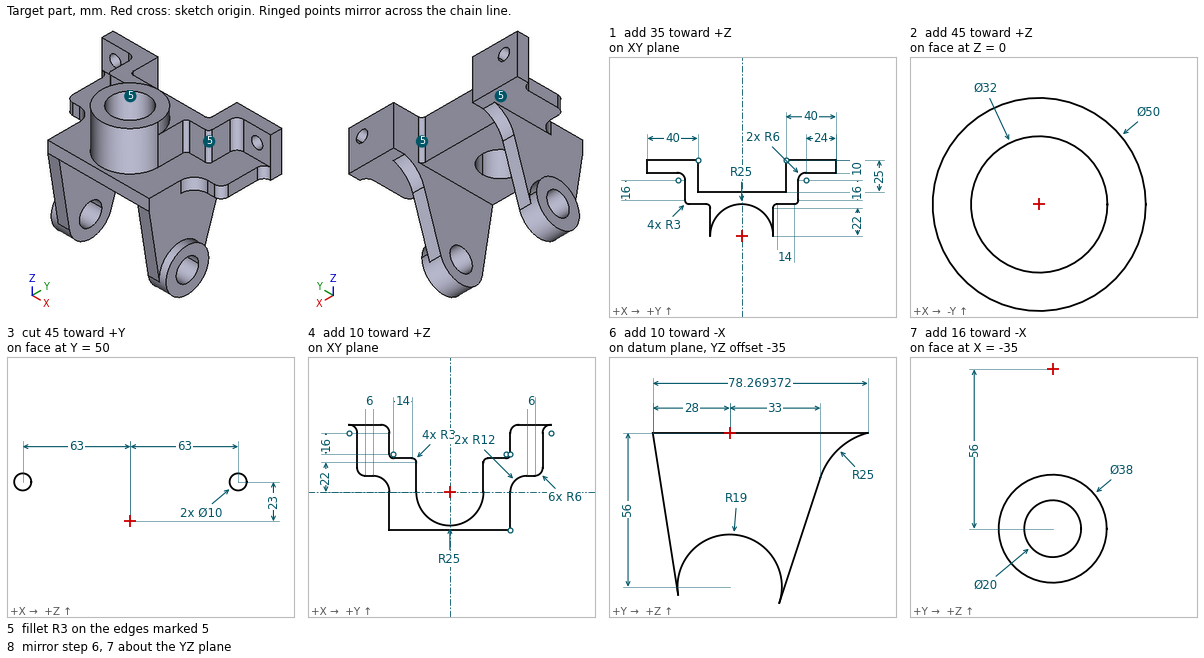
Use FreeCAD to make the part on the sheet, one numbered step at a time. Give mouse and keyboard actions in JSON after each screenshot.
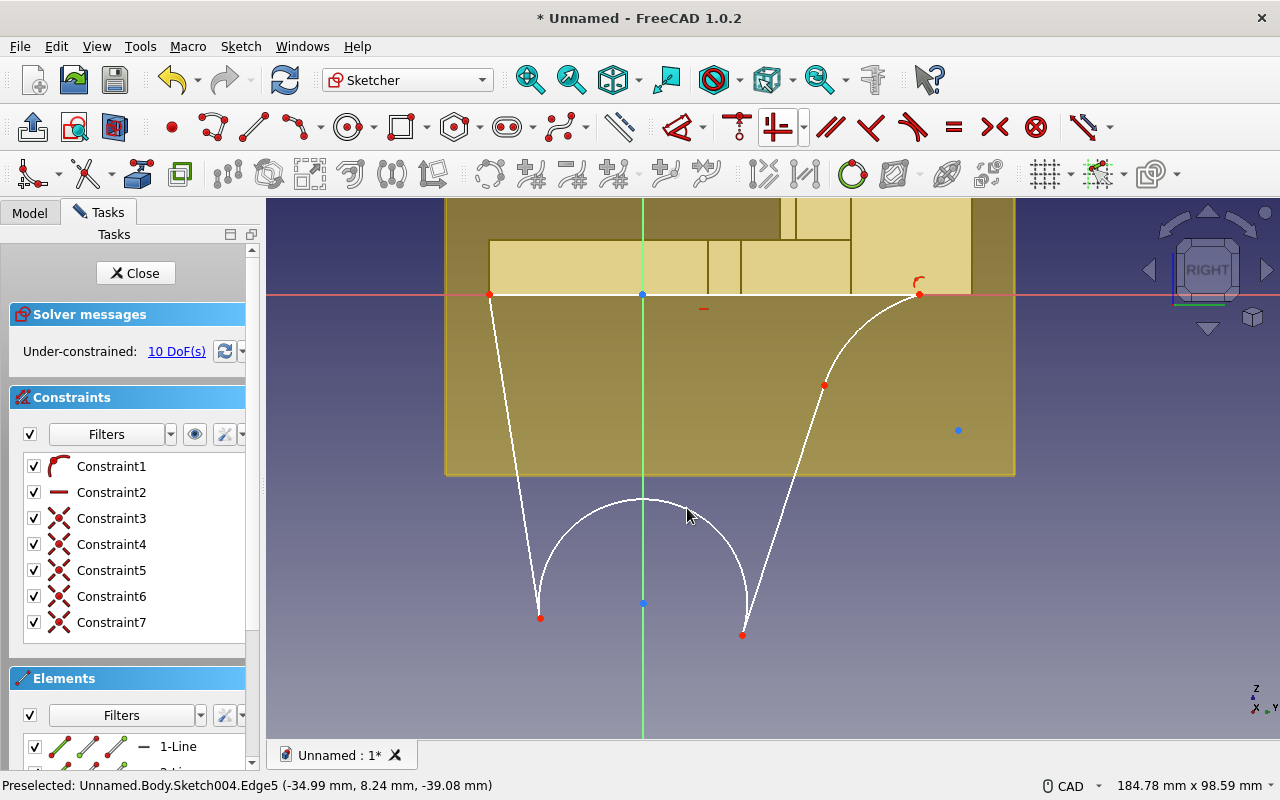
{"action": "left_click", "coordinate": [767, 561]}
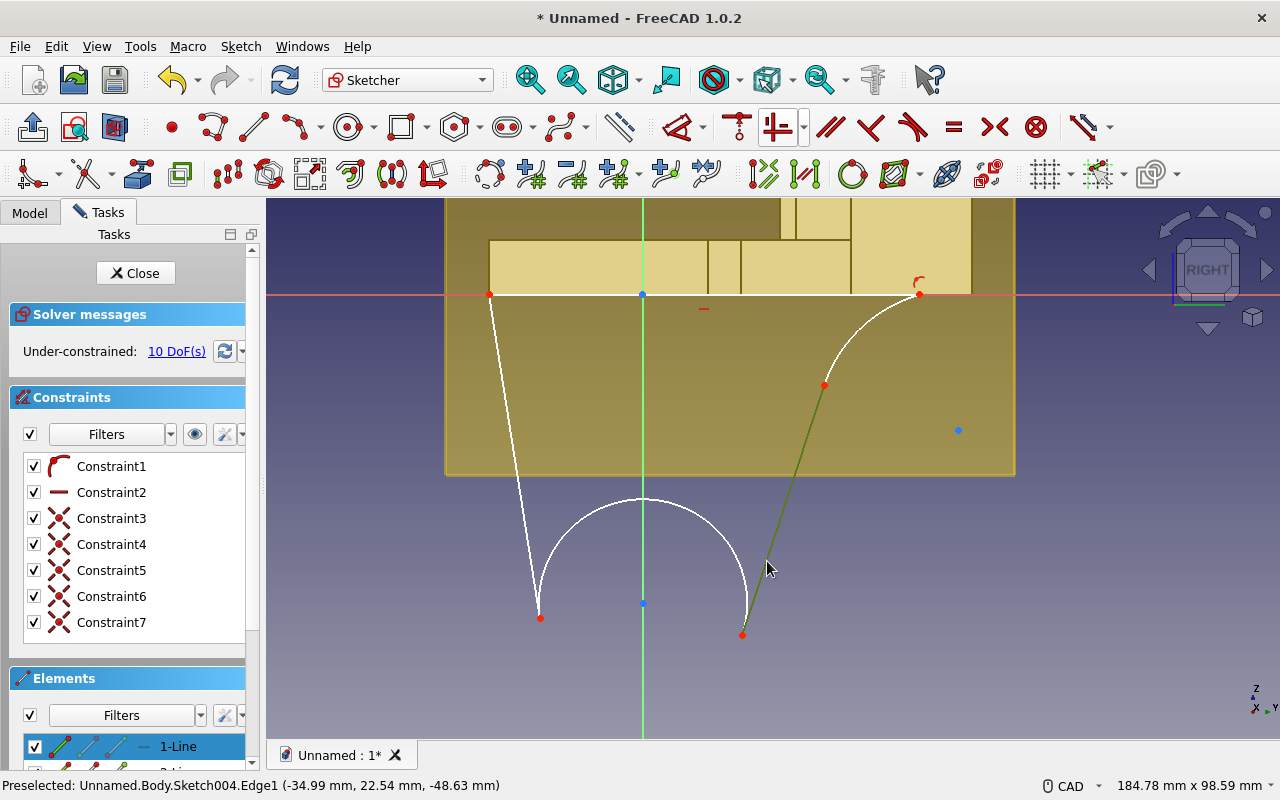
{"action": "left_click", "coordinate": [882, 312]}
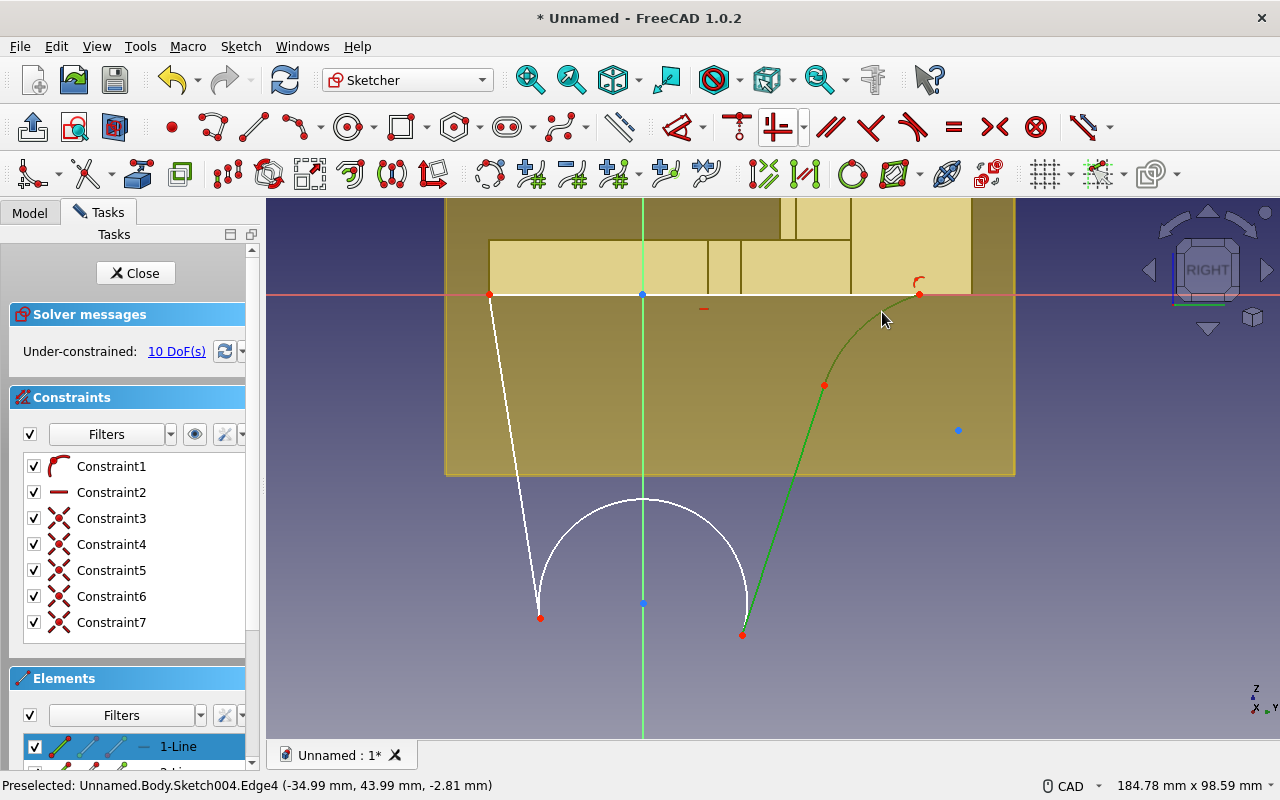
{"action": "left_click", "coordinate": [913, 128]}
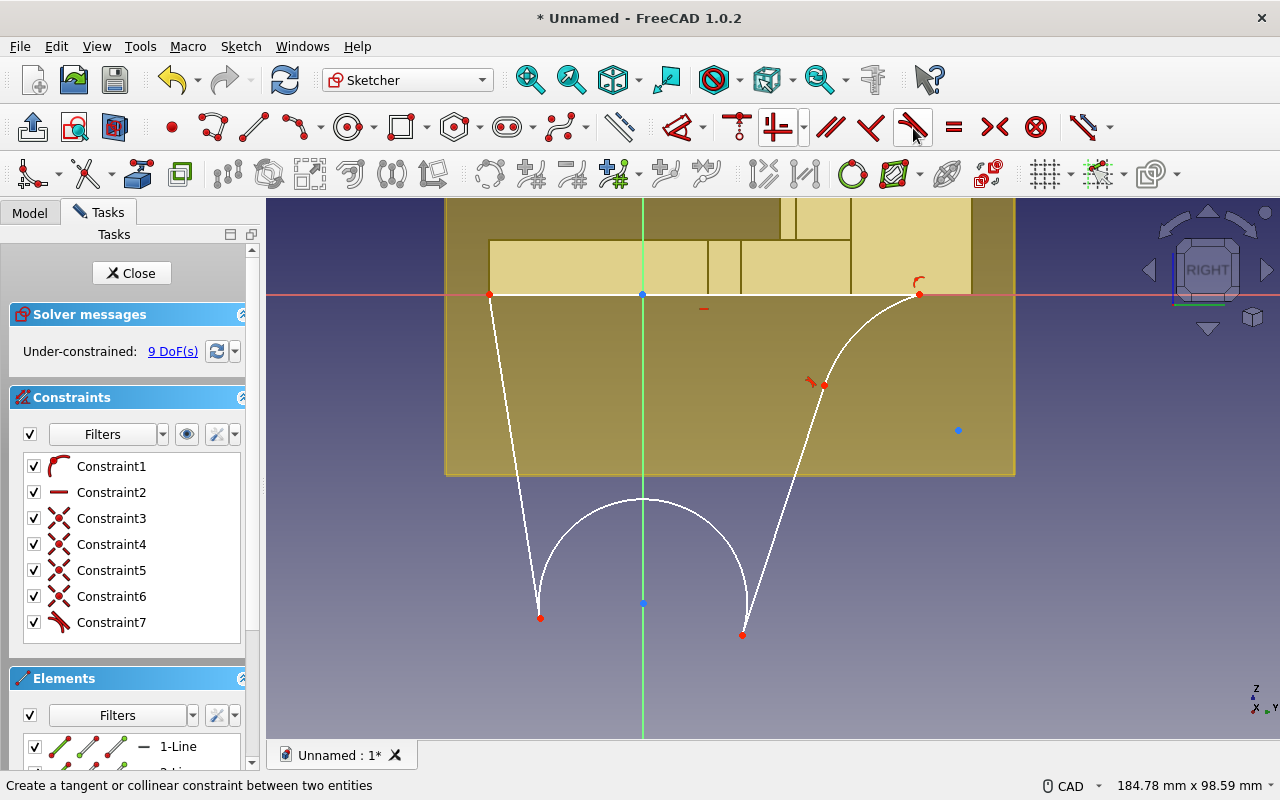
{"action": "left_click", "coordinate": [767, 561]}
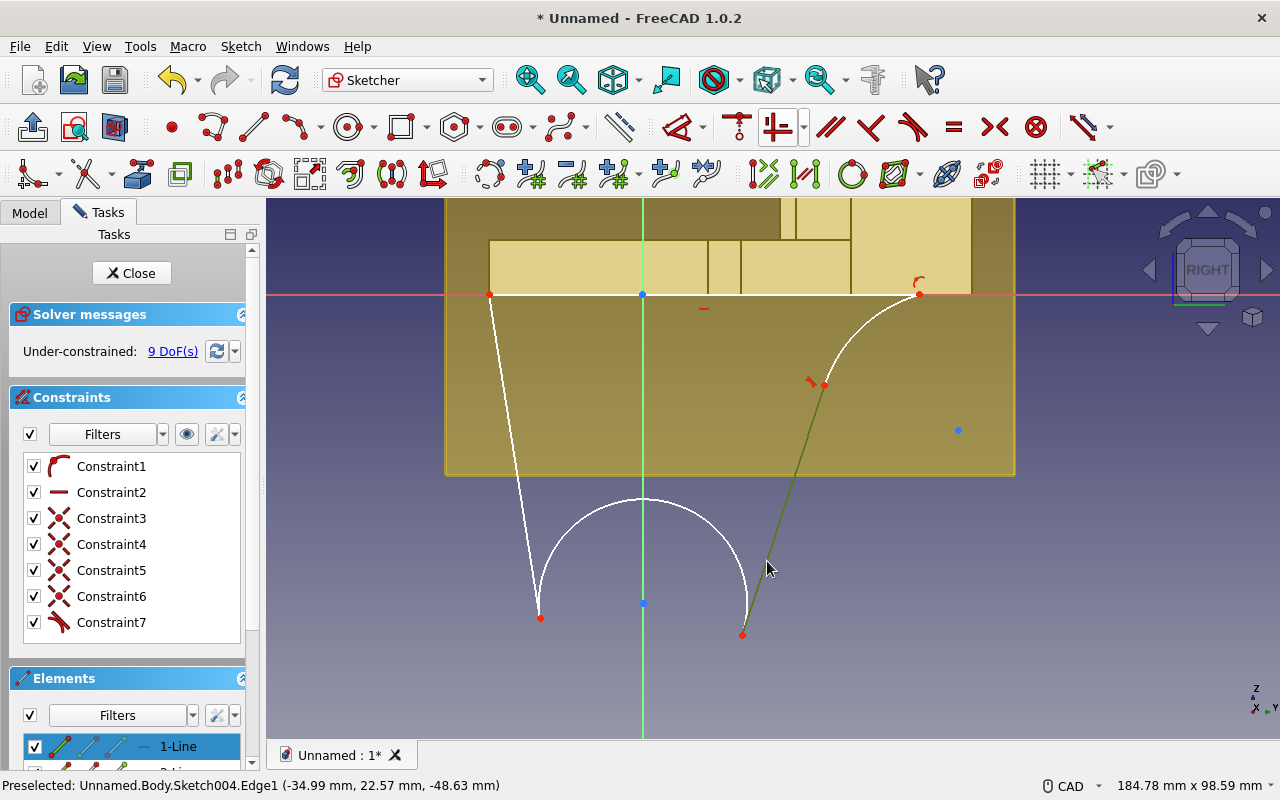
{"action": "left_click", "coordinate": [718, 531]}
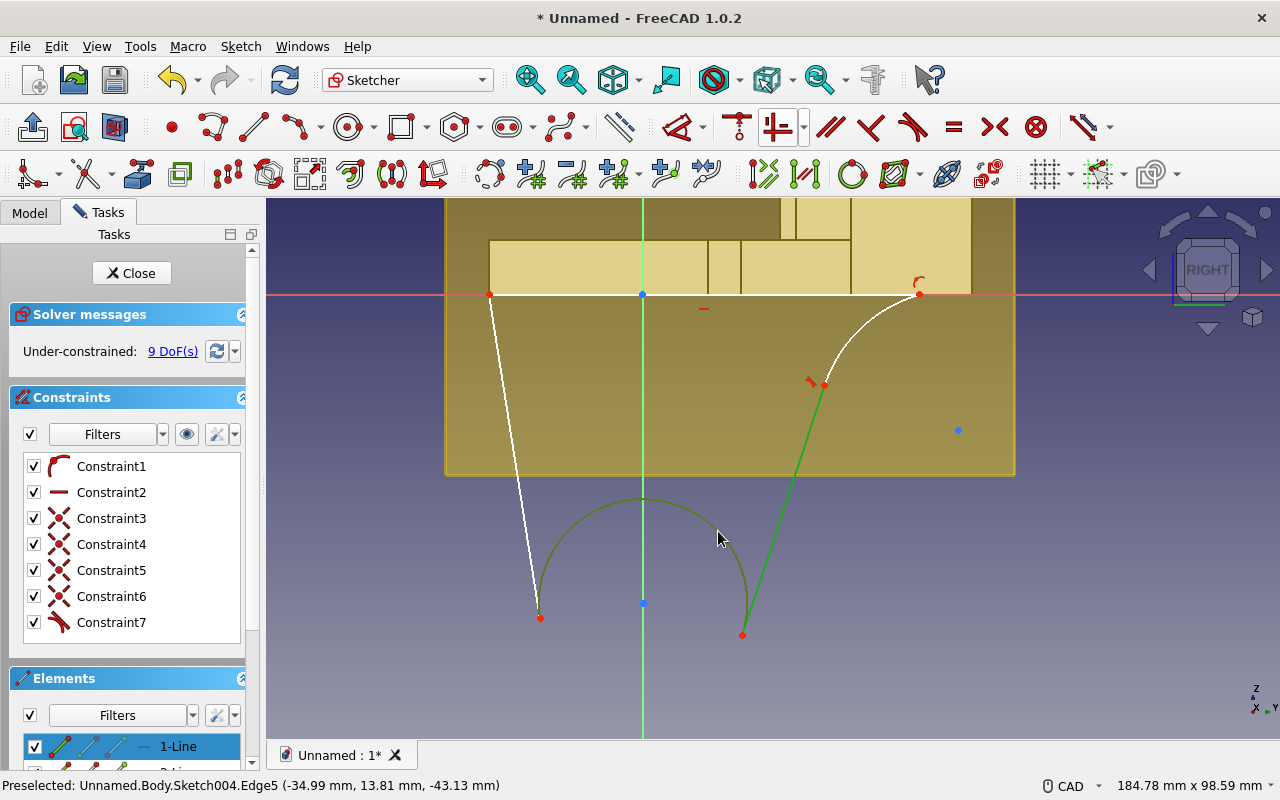
{"action": "left_click", "coordinate": [913, 128]}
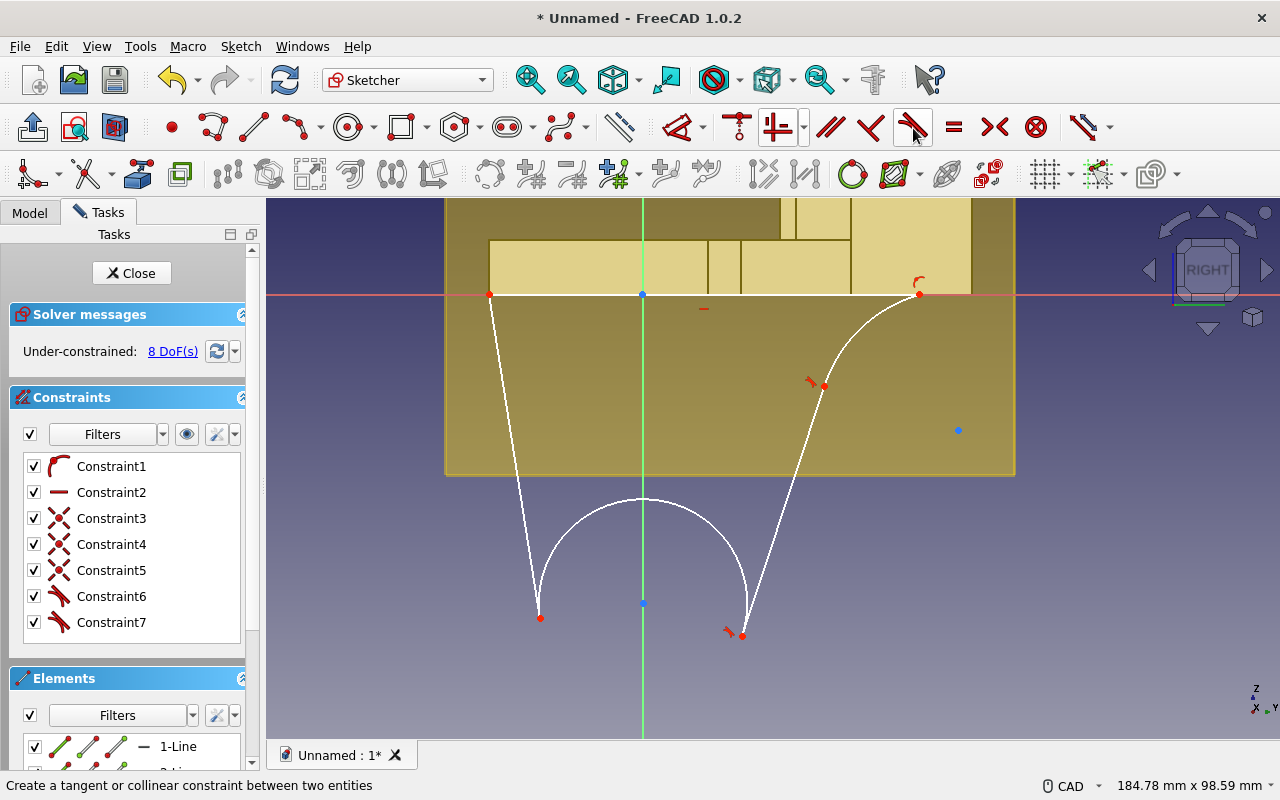
{"action": "left_click", "coordinate": [504, 392]}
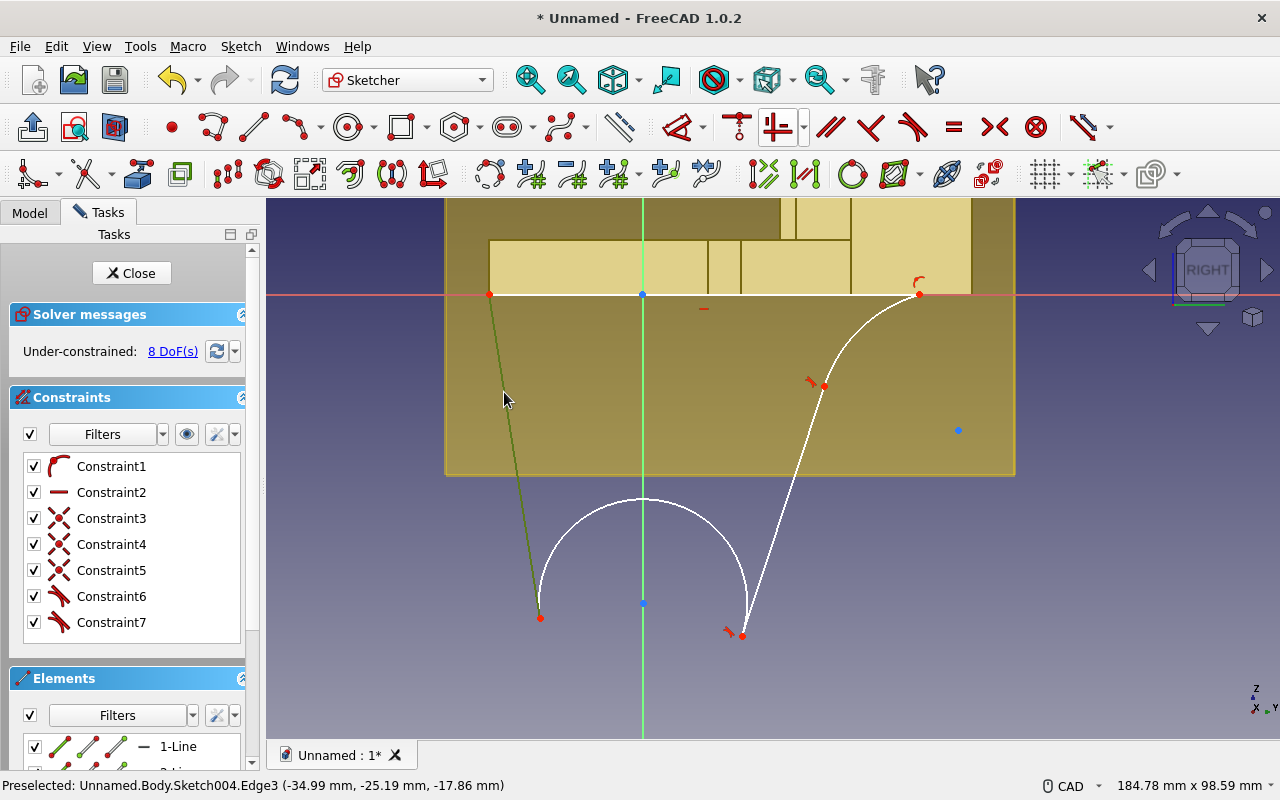
{"action": "left_click", "coordinate": [718, 531]}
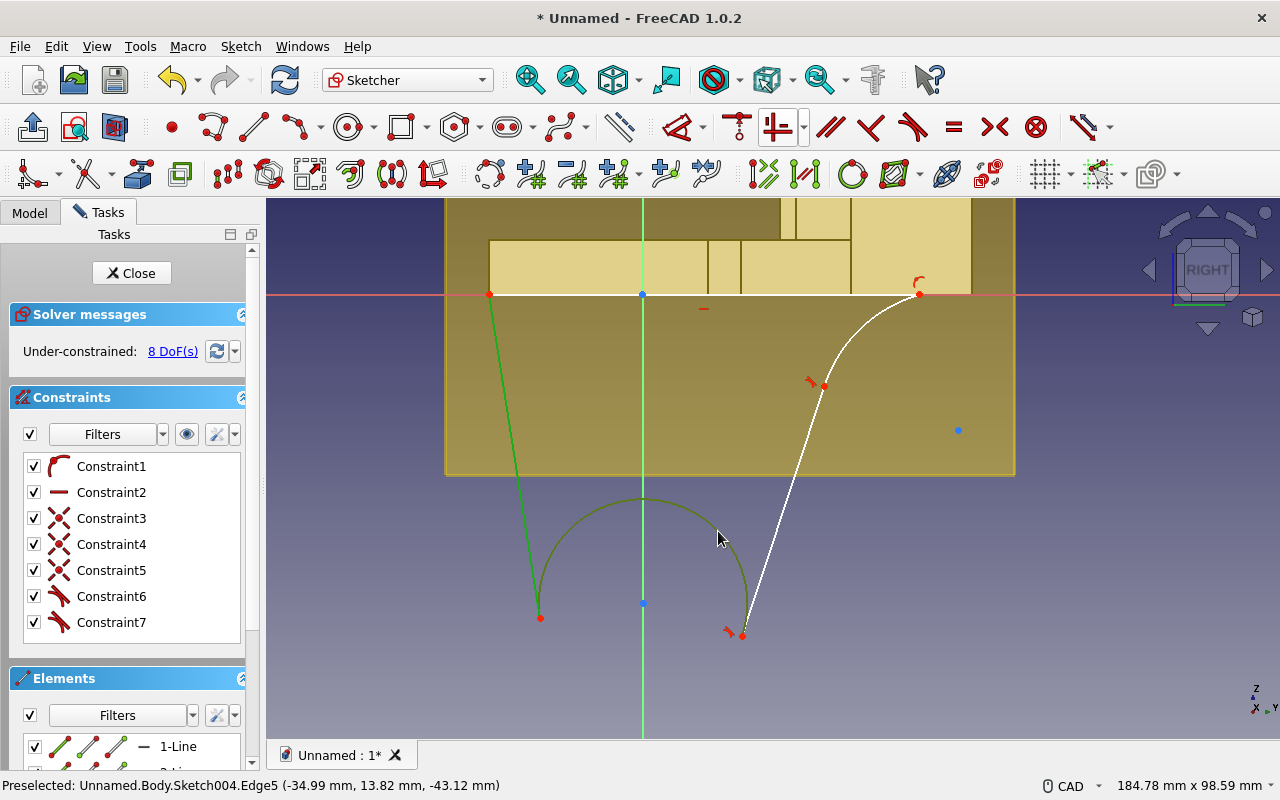
{"action": "left_click", "coordinate": [913, 128]}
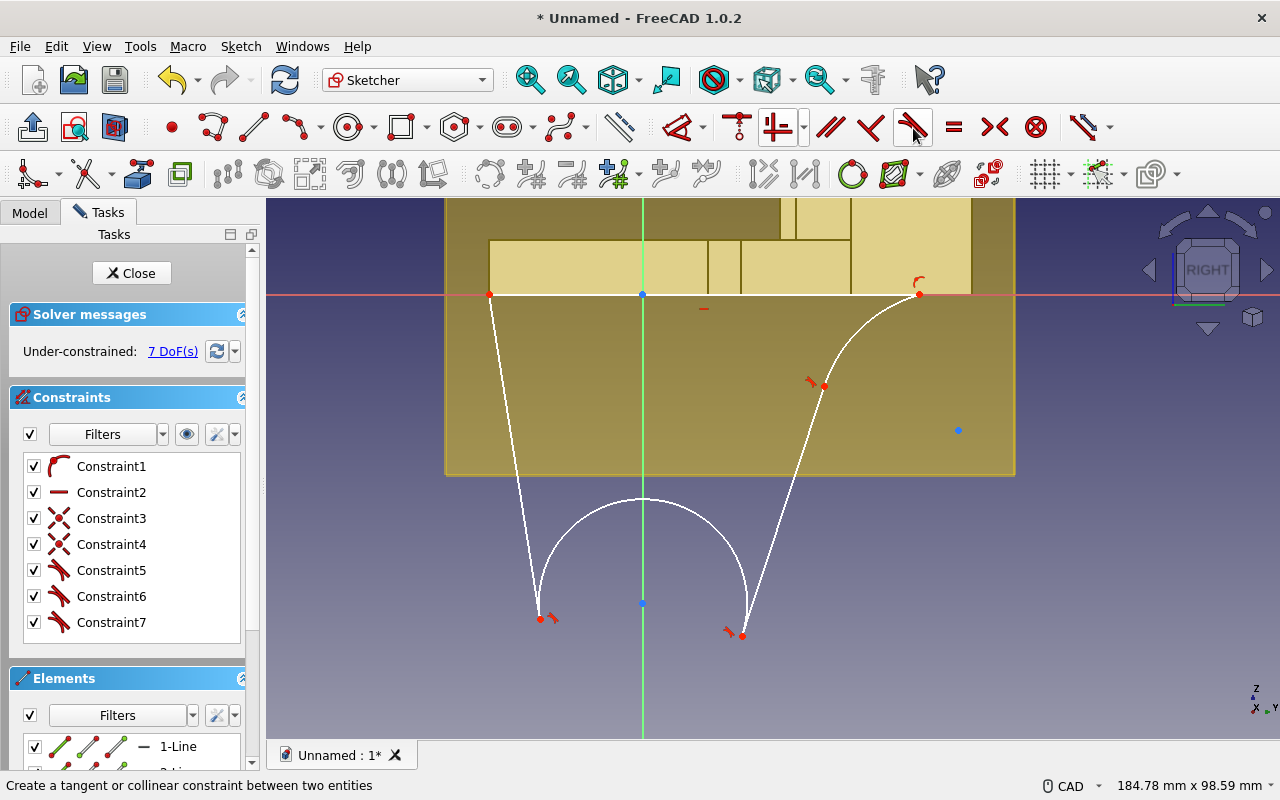
{"action": "left_click", "coordinate": [643, 603]}